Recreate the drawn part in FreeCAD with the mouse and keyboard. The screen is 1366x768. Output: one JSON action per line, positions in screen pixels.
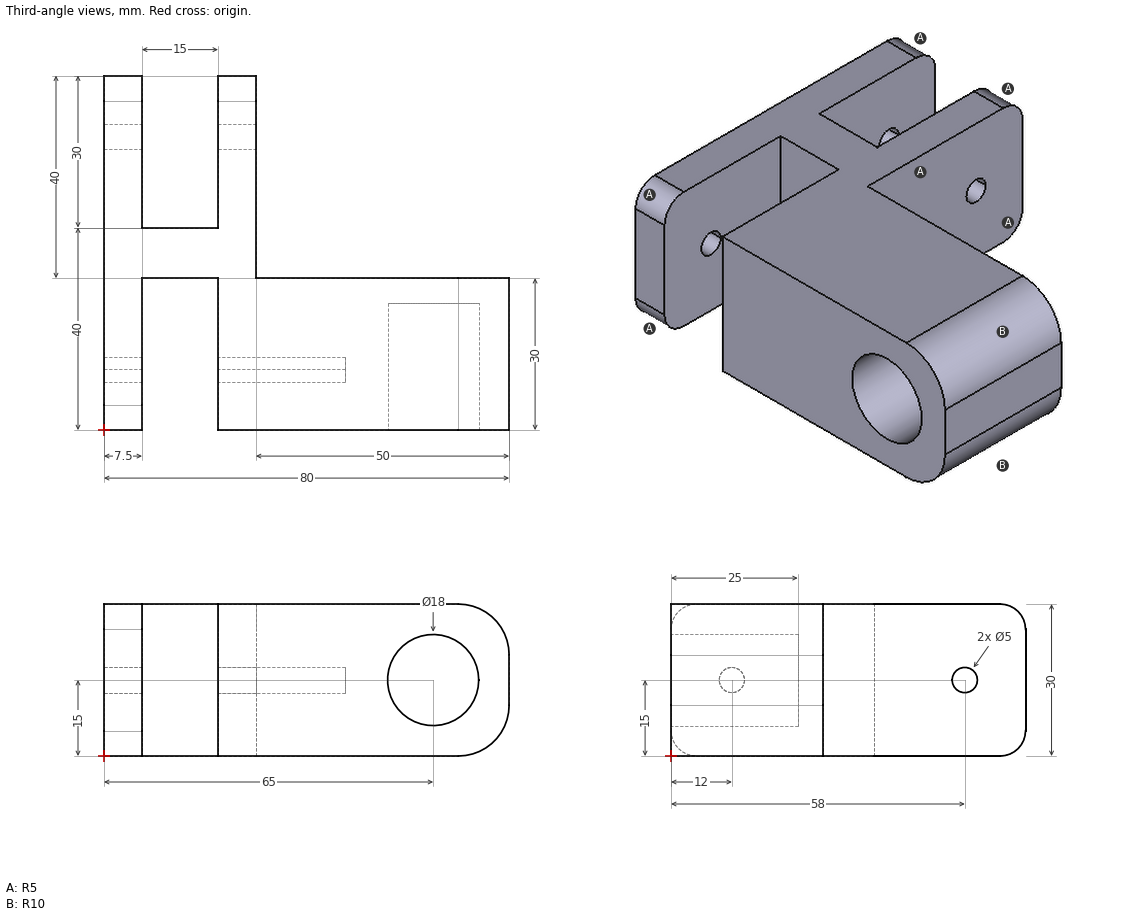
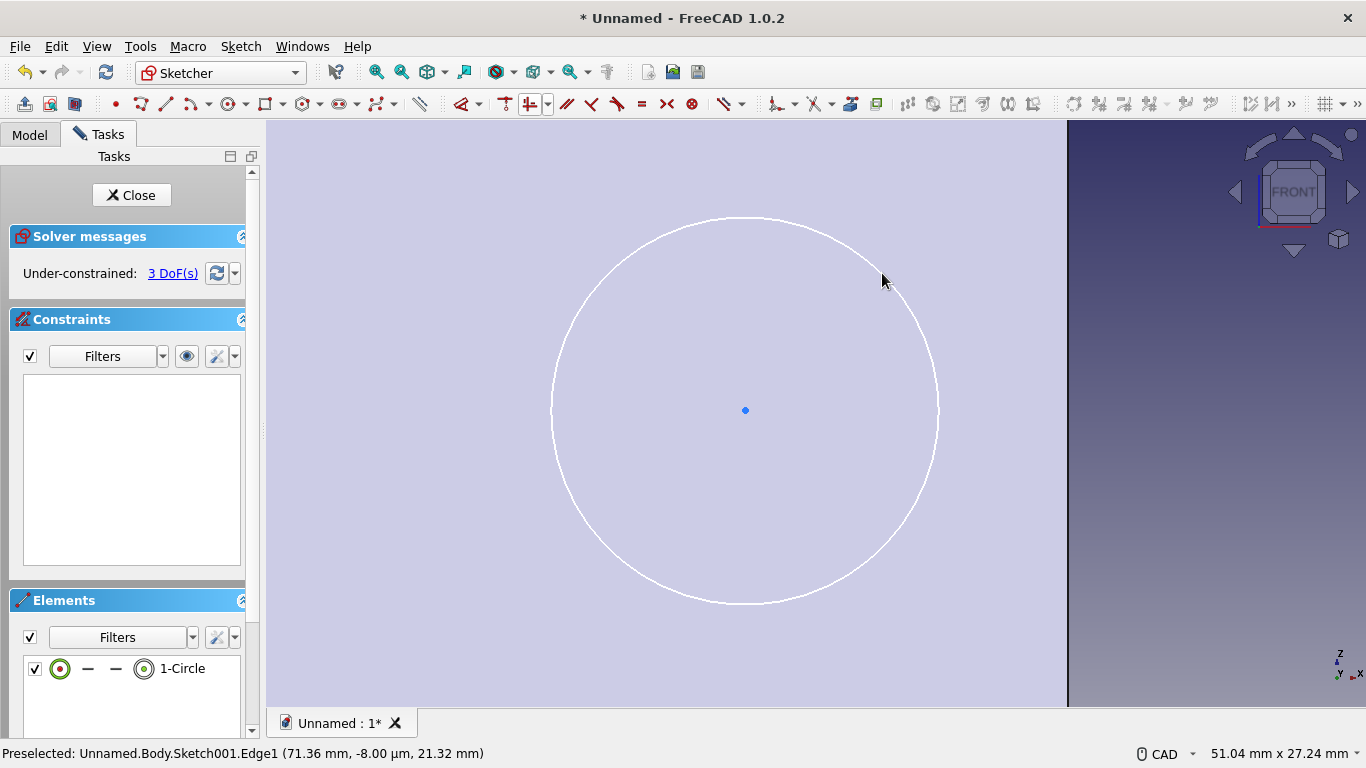
{"action": "left_click", "coordinate": [460, 104]}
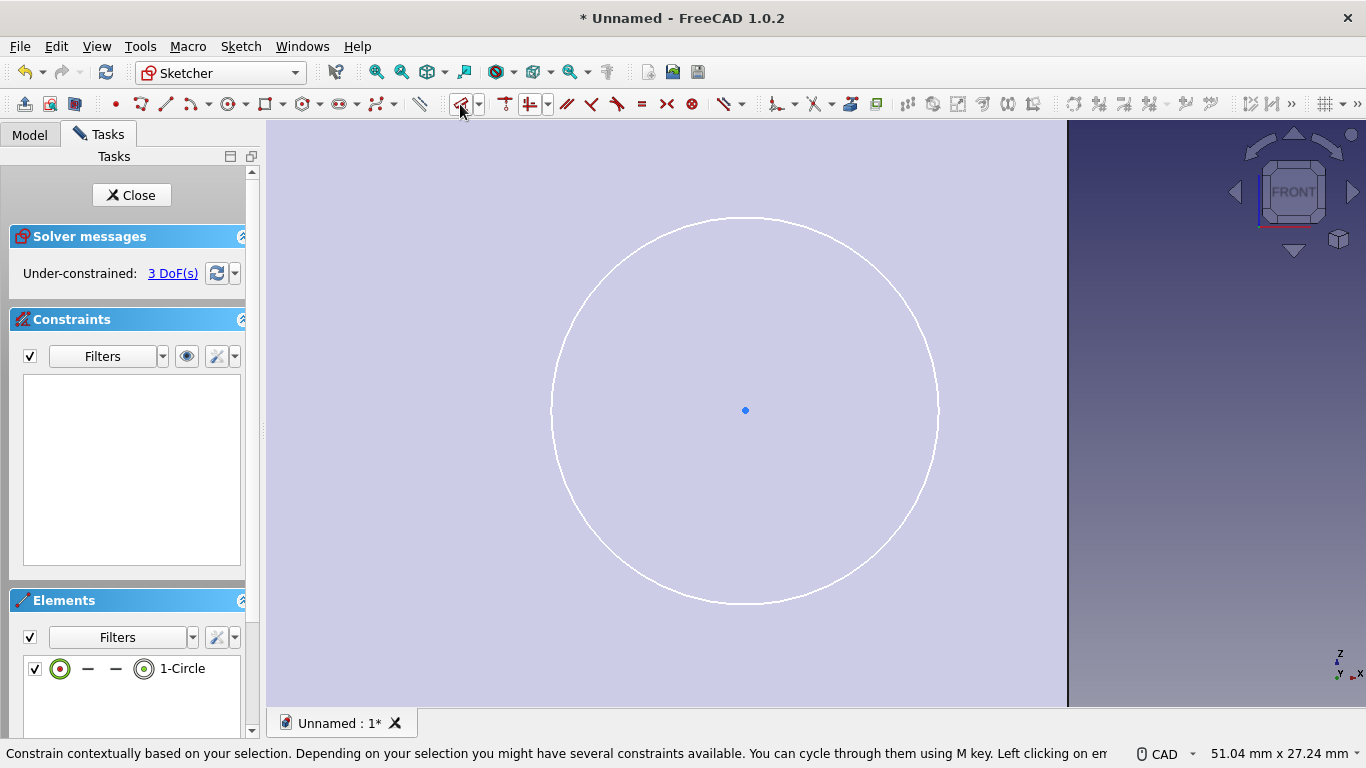
{"action": "left_click", "coordinate": [882, 274]}
{"action": "left_click", "coordinate": [905, 251]}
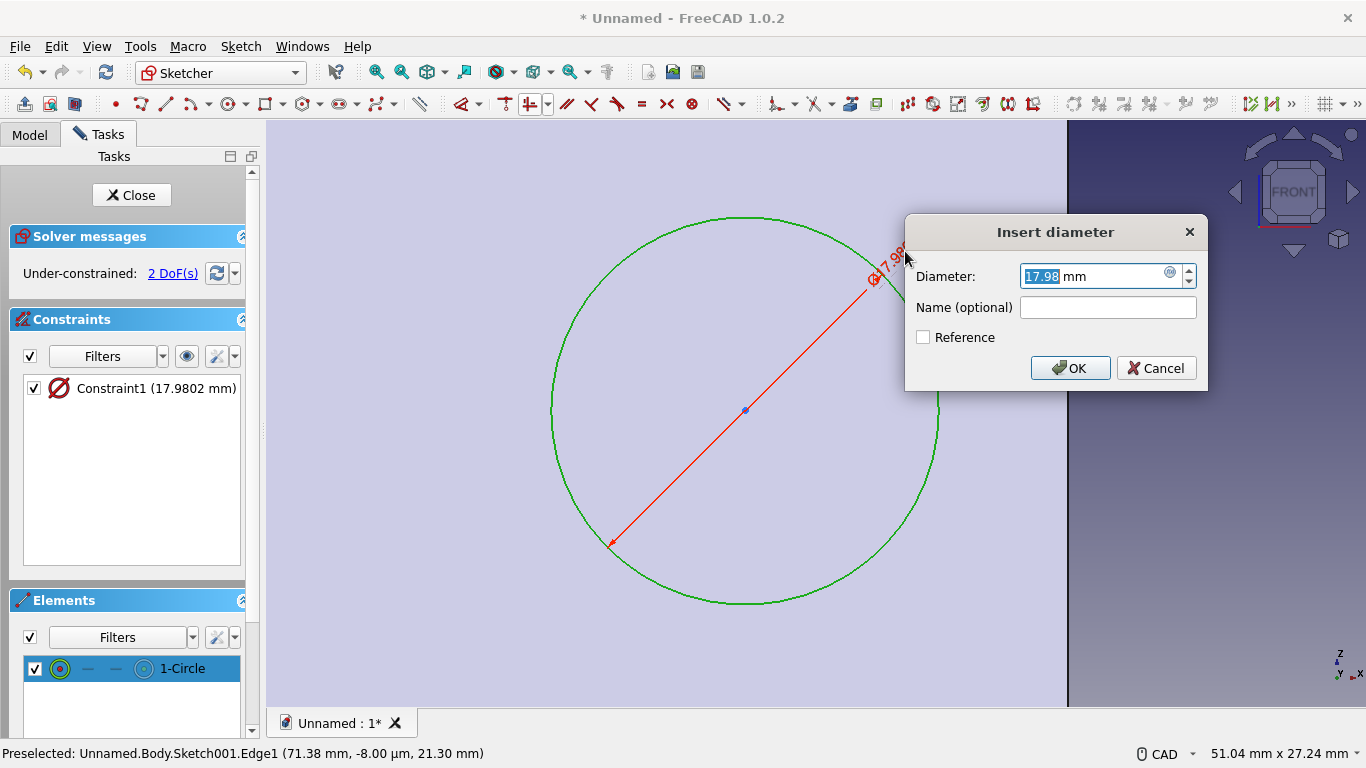
{"action": "type", "text": "18"}
{"action": "key", "text": "Return"}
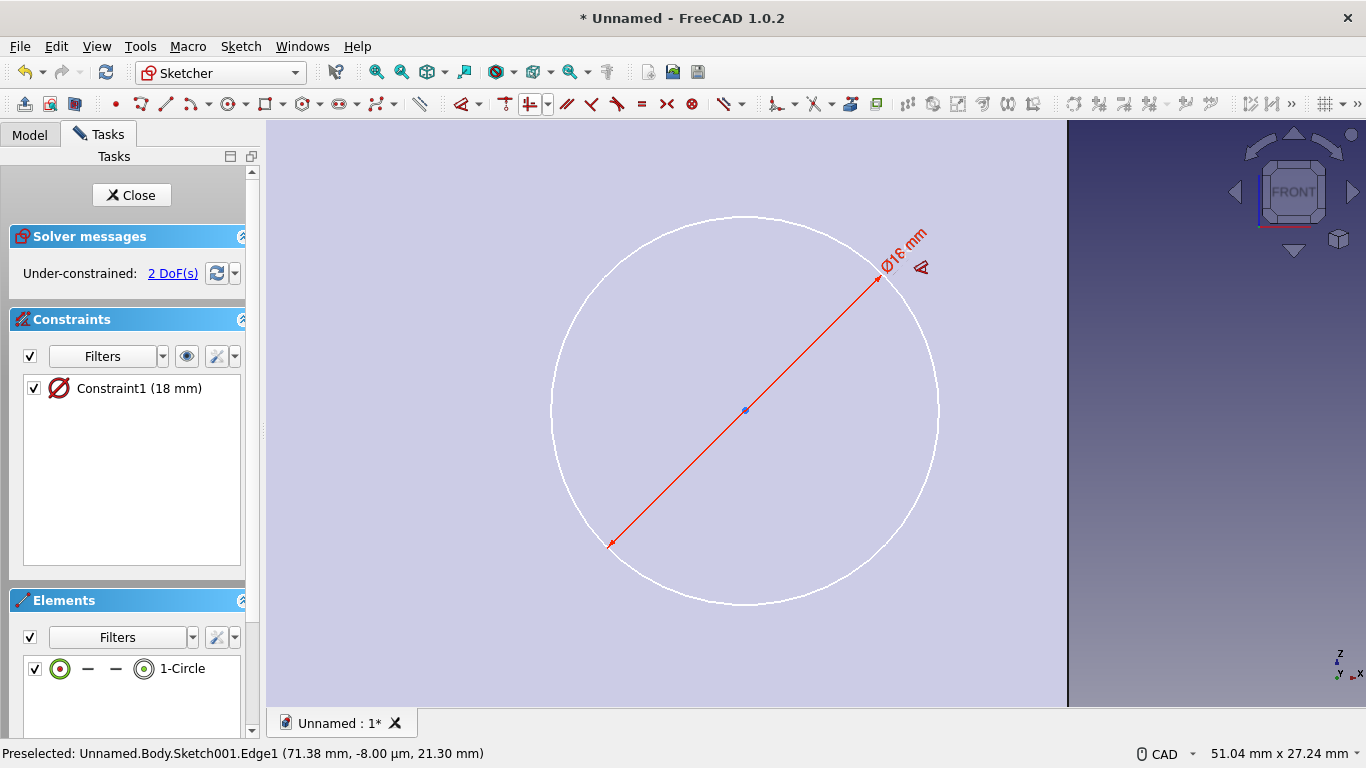
{"action": "left_click", "coordinate": [745, 411]}
{"action": "left_click", "coordinate": [520, 377]}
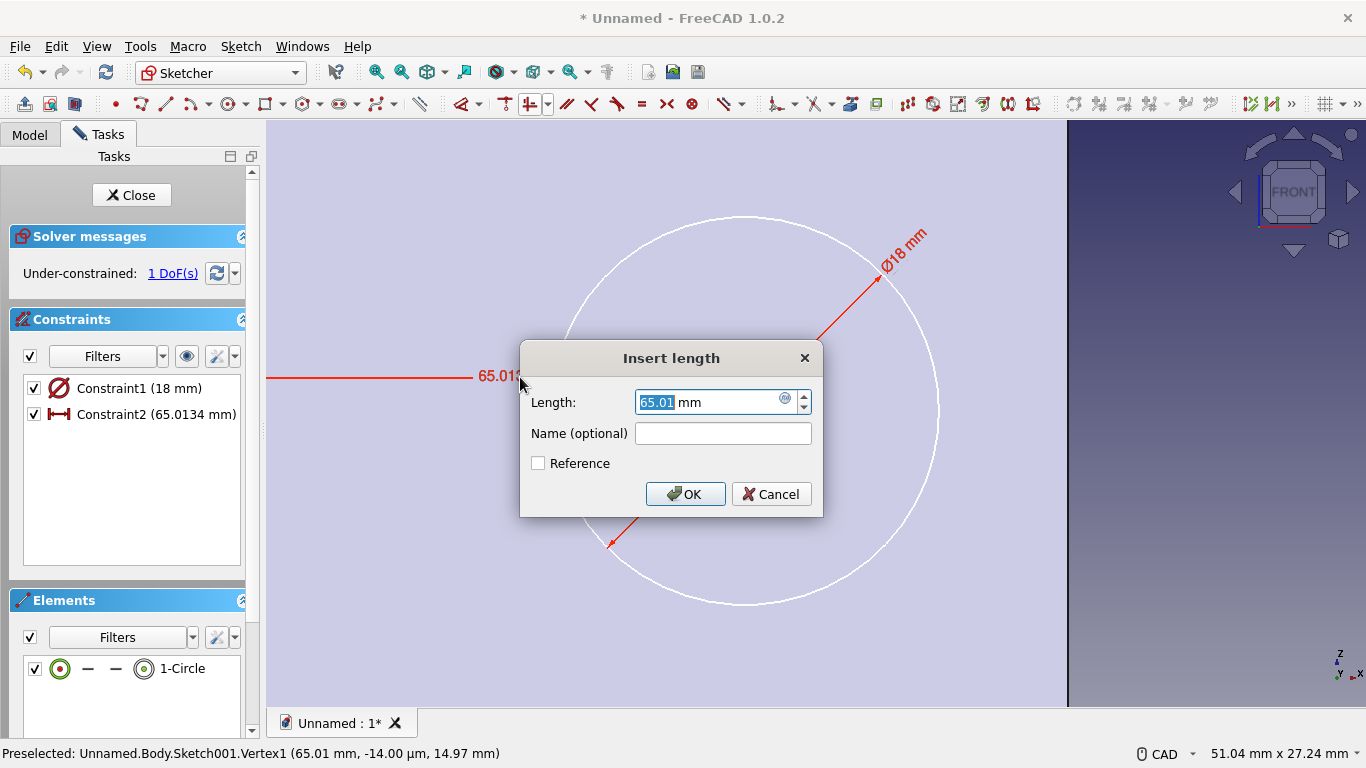
{"action": "type", "text": "65"}
{"action": "key", "text": "Return"}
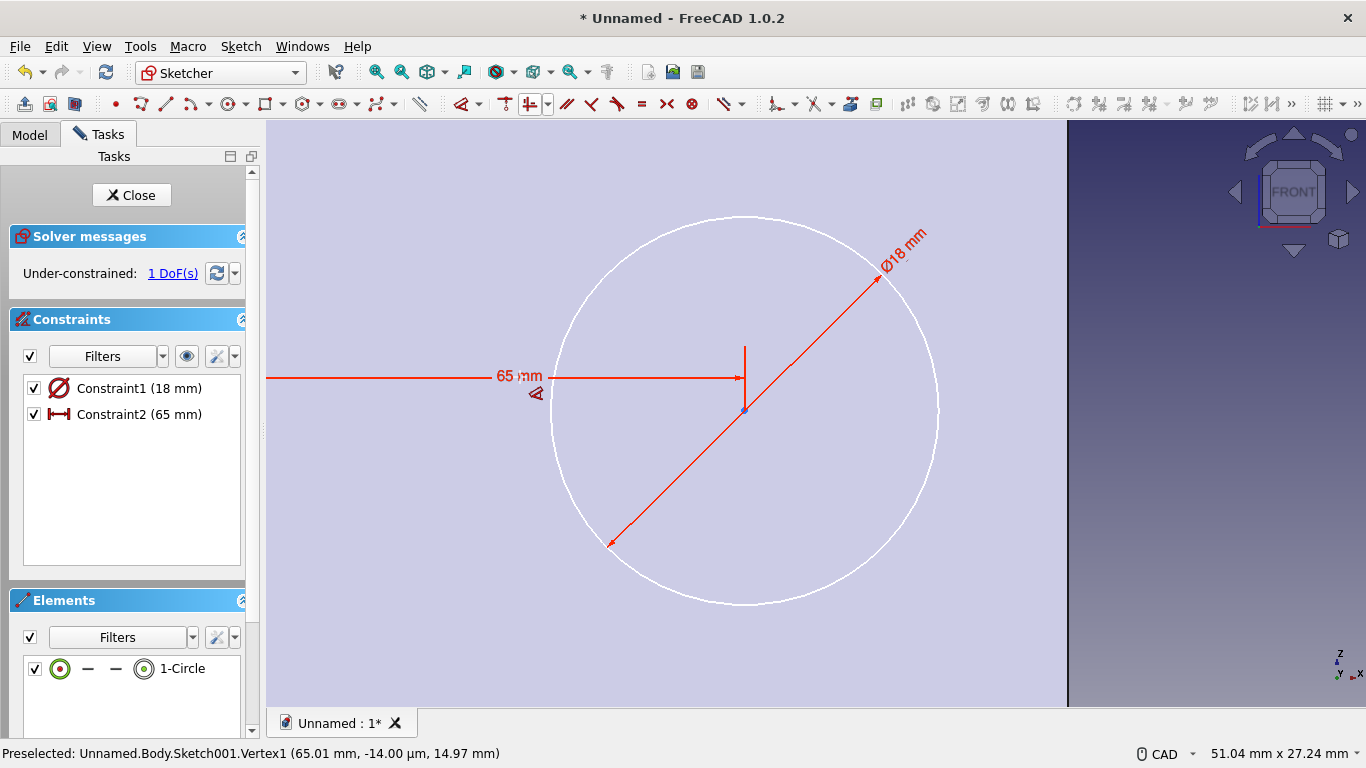
{"action": "left_click", "coordinate": [745, 411]}
{"action": "left_click", "coordinate": [779, 545]}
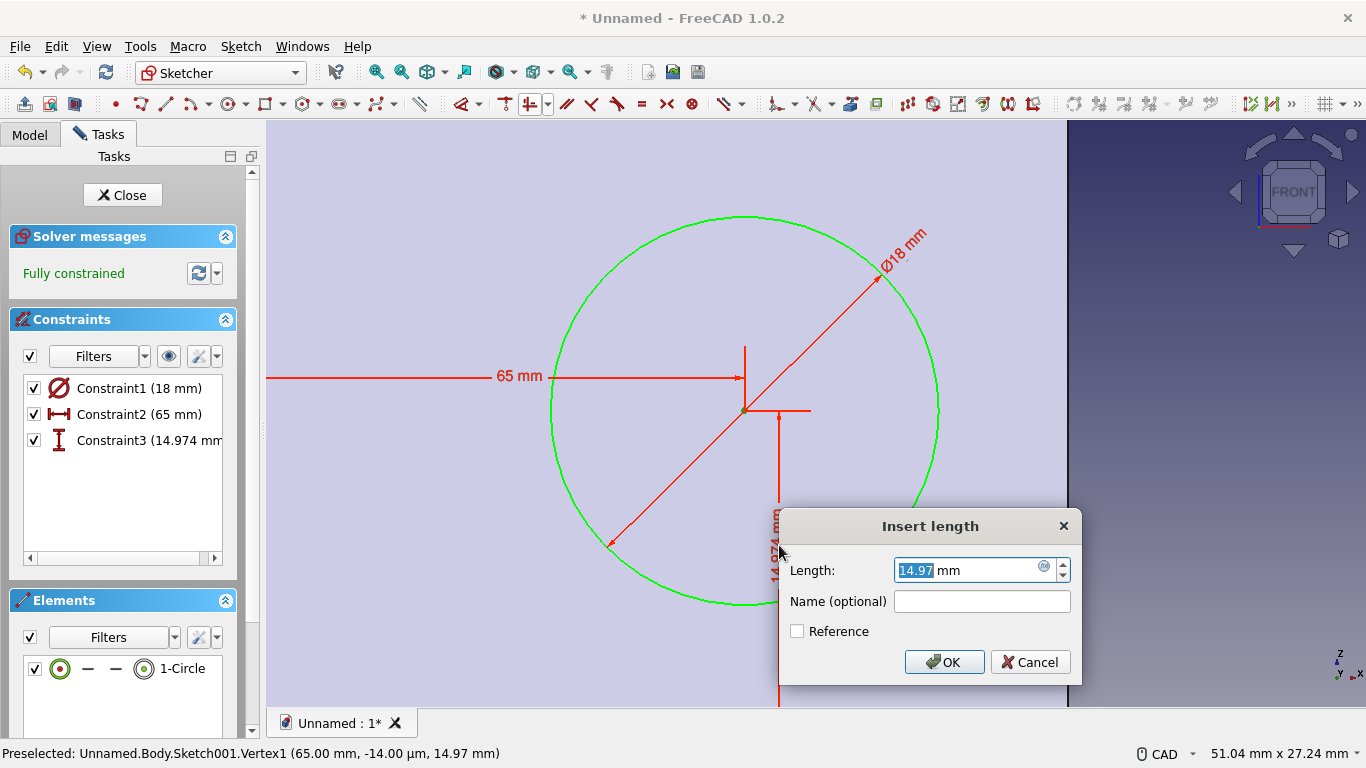
{"action": "type", "text": "15"}
{"action": "key", "text": "Return"}
{"action": "key", "text": "Escape"}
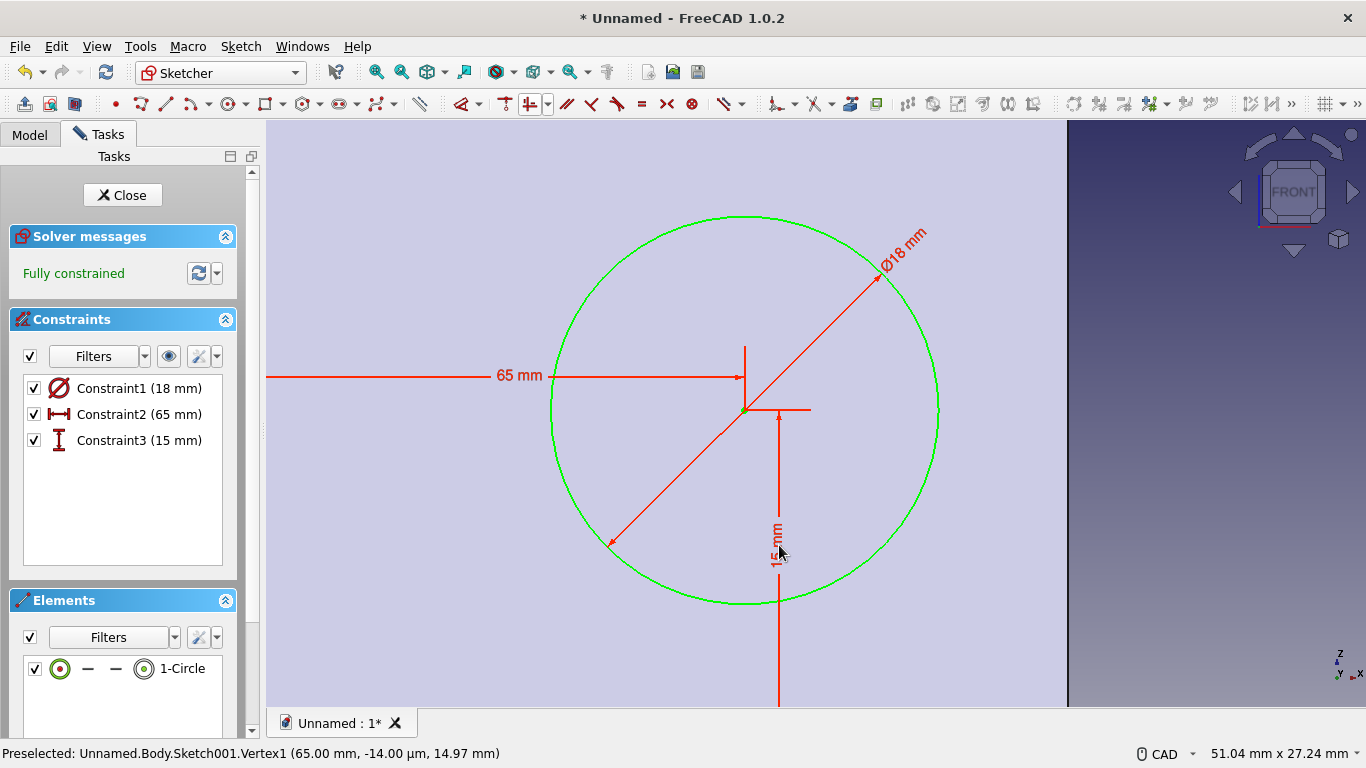
{"action": "left_click", "coordinate": [123, 195]}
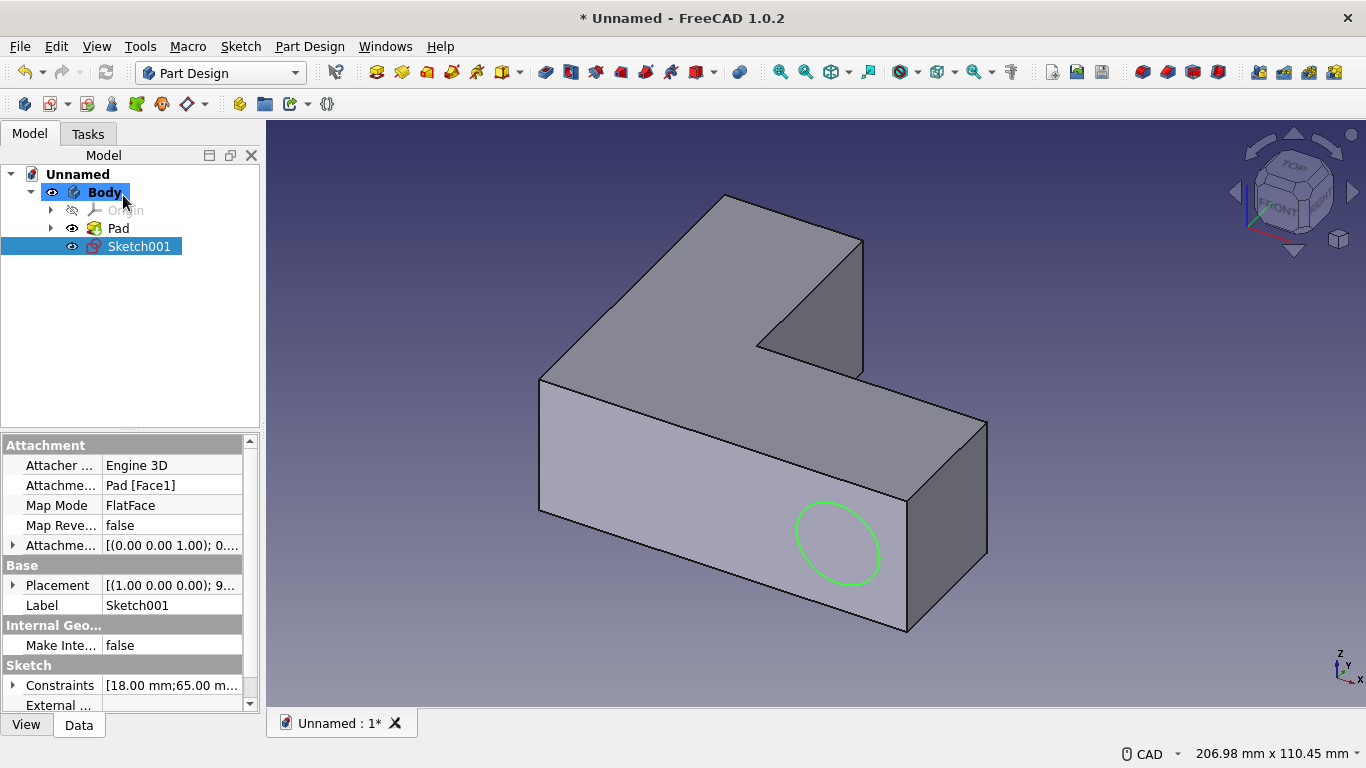
{"action": "left_click", "coordinate": [546, 72]}